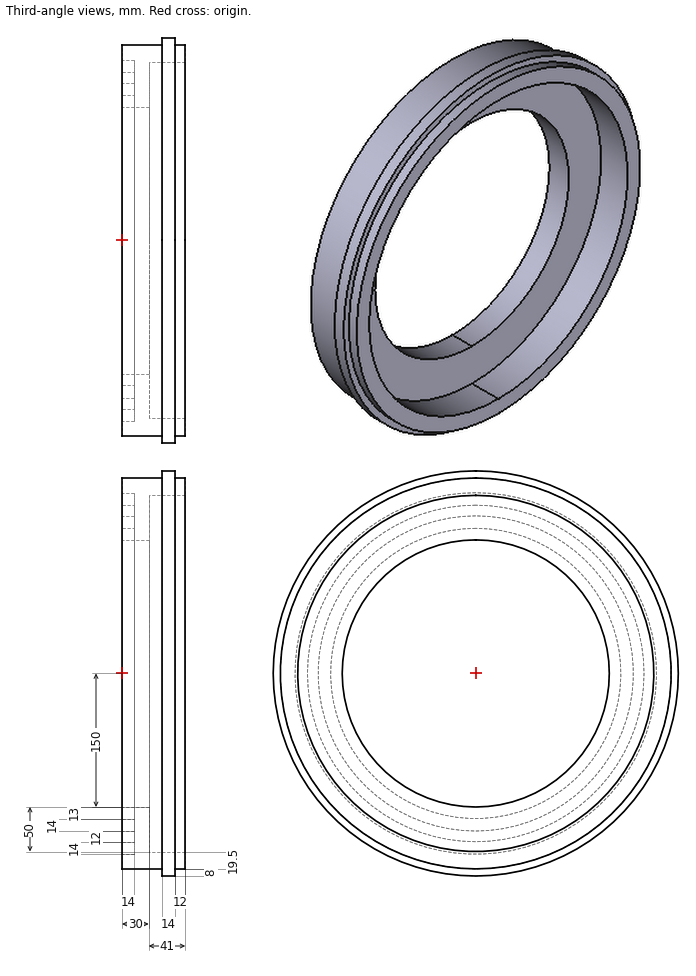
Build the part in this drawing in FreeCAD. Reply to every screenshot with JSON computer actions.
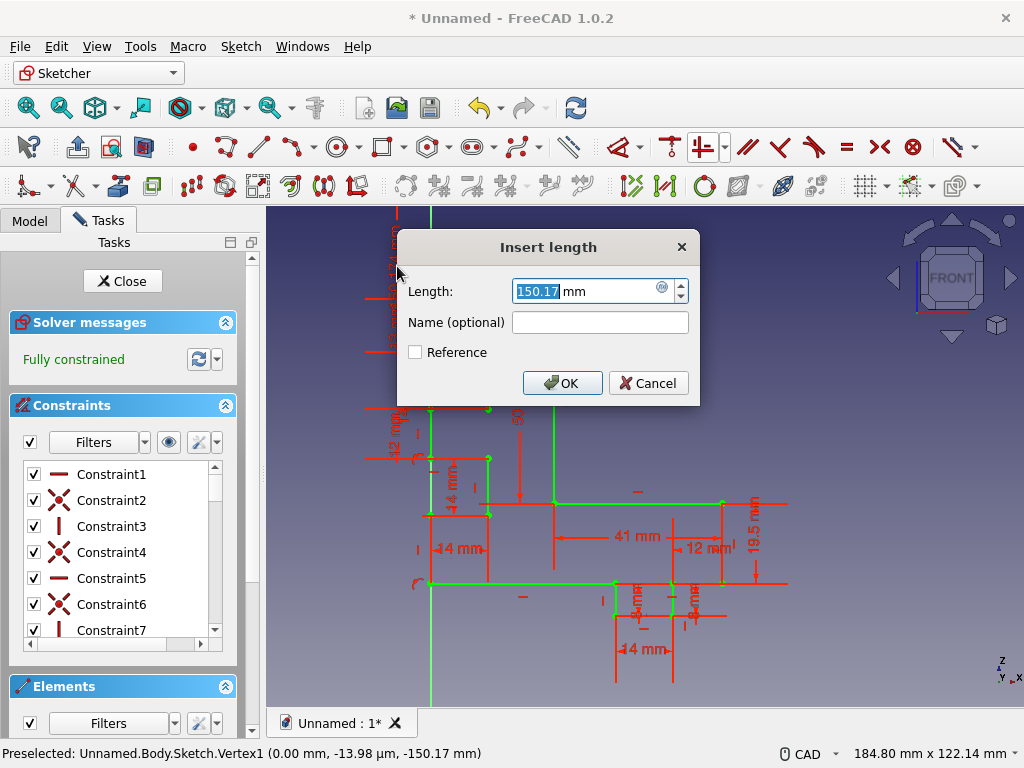
{"action": "type", "text": "150"}
{"action": "key", "text": "Return"}
{"action": "key", "text": "Escape"}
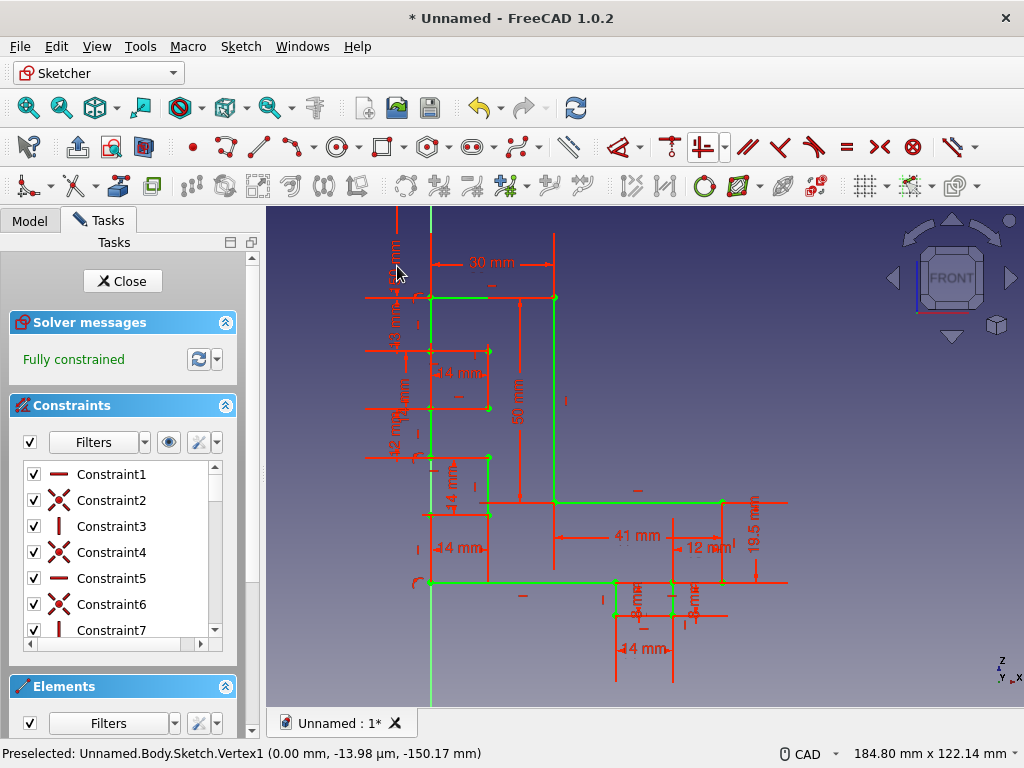
{"action": "left_click", "coordinate": [123, 281]}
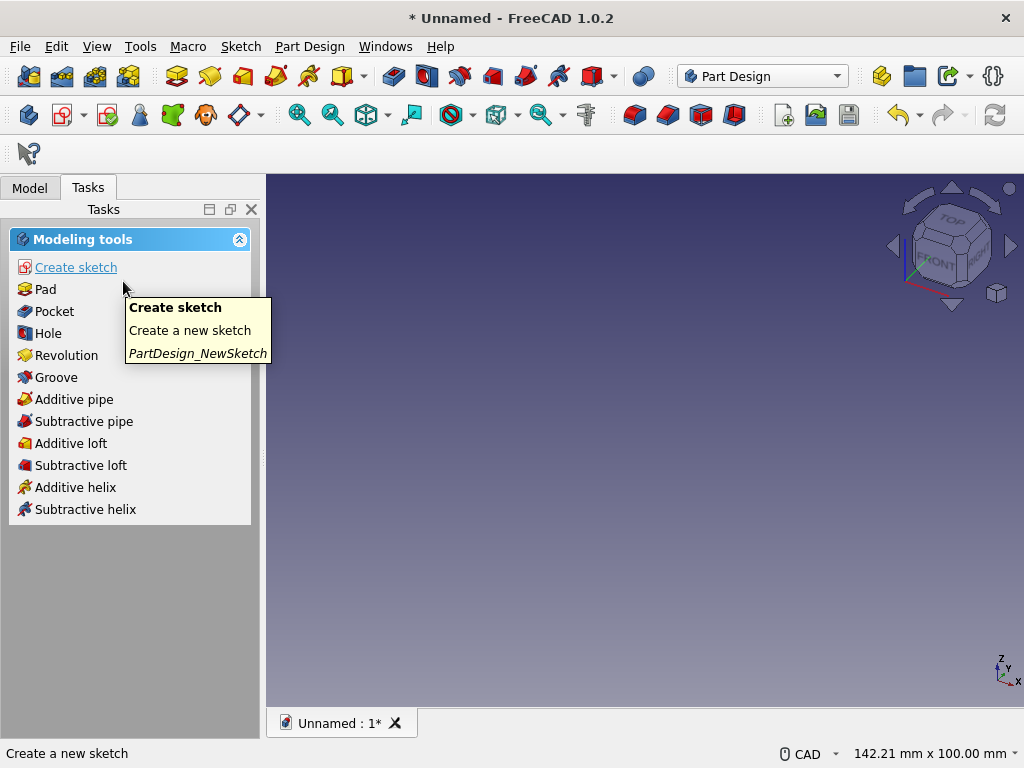
{"action": "left_click", "coordinate": [210, 76]}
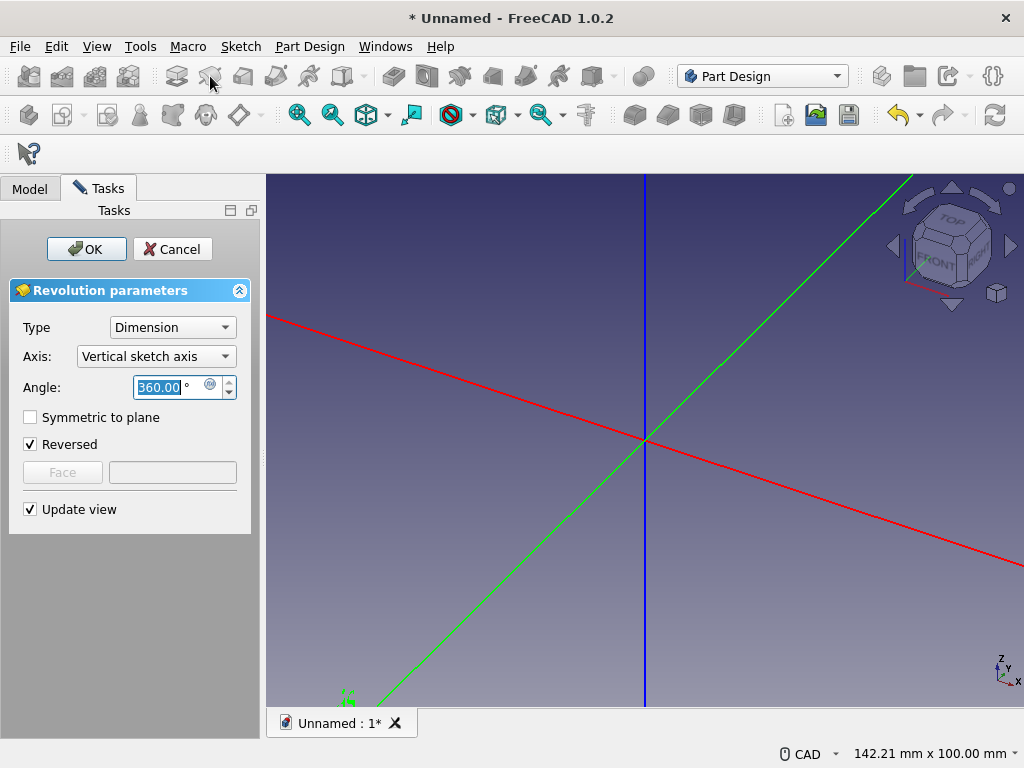
{"action": "left_click", "coordinate": [157, 356]}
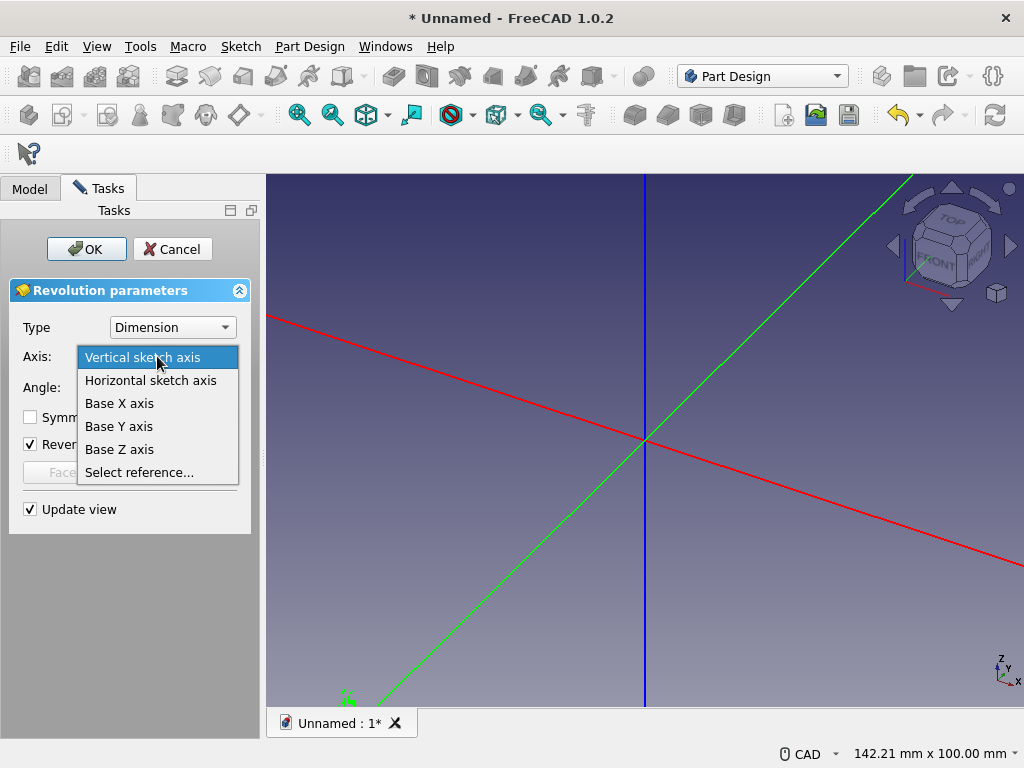
{"action": "left_click", "coordinate": [156, 380]}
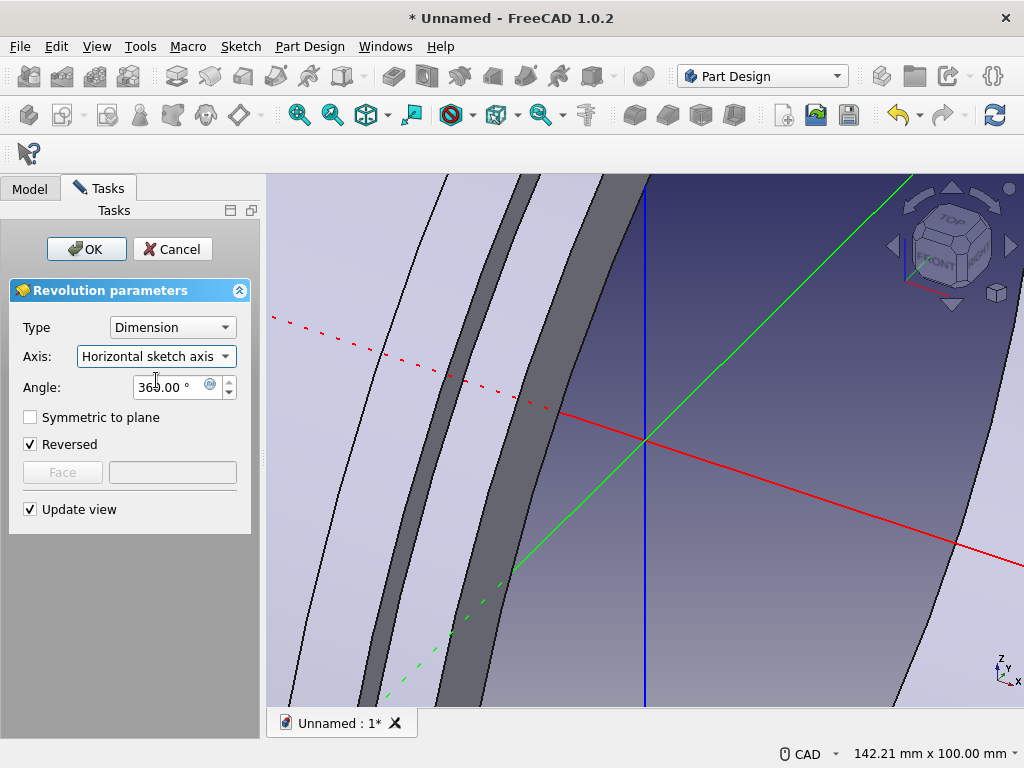
{"action": "left_click", "coordinate": [87, 249]}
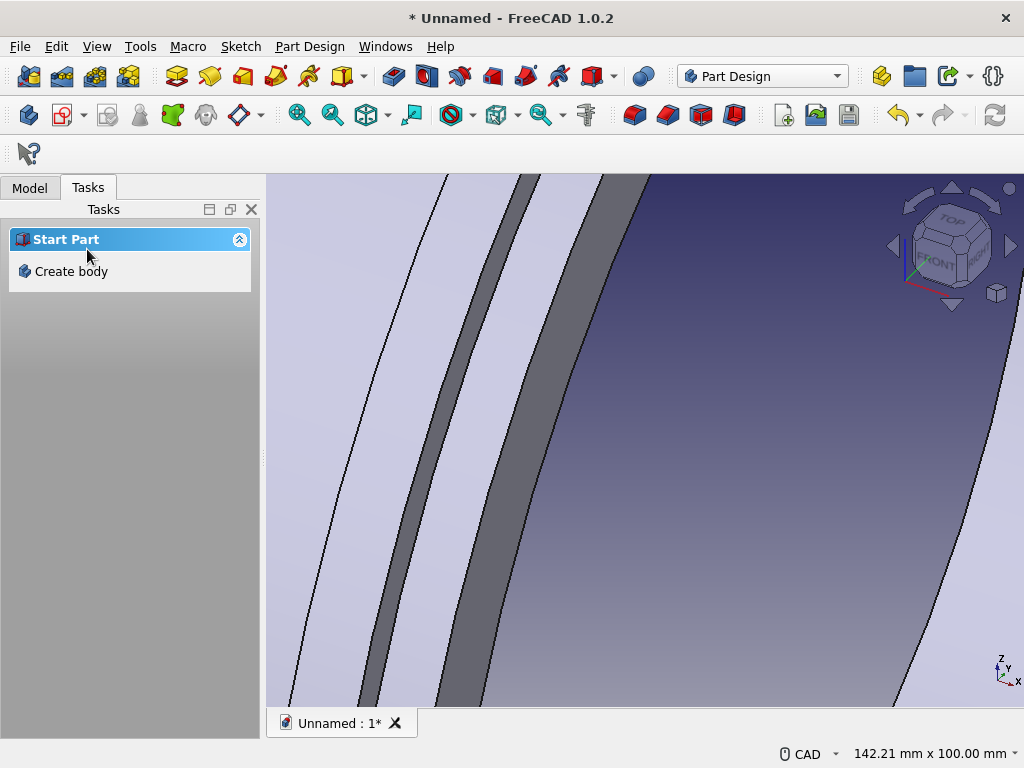
{"action": "key", "text": "0"}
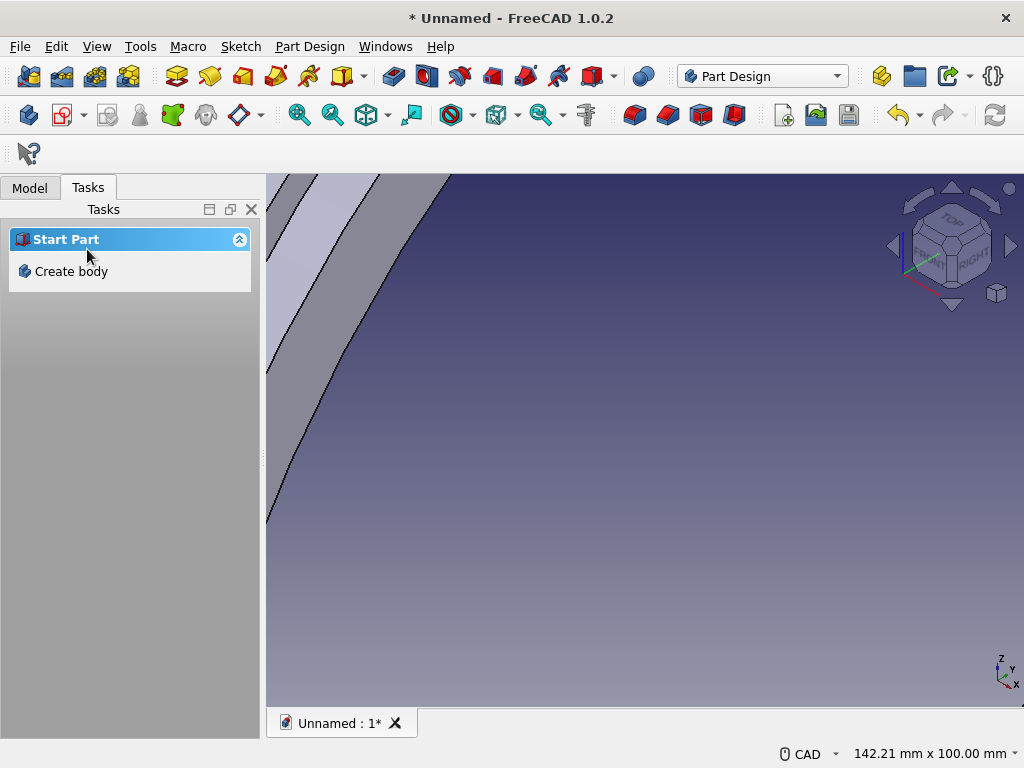
{"action": "left_click", "coordinate": [300, 116]}